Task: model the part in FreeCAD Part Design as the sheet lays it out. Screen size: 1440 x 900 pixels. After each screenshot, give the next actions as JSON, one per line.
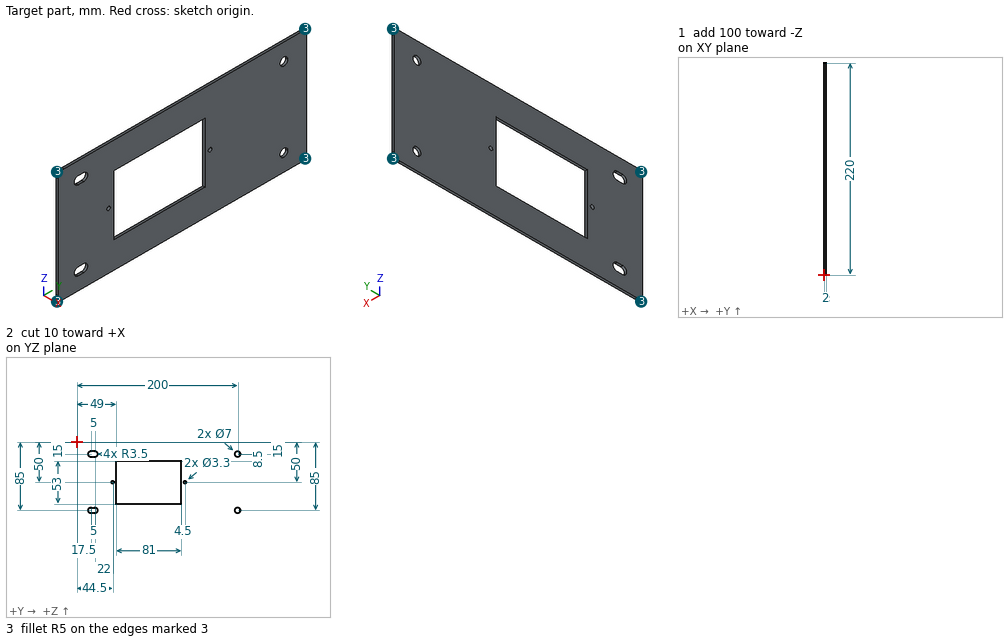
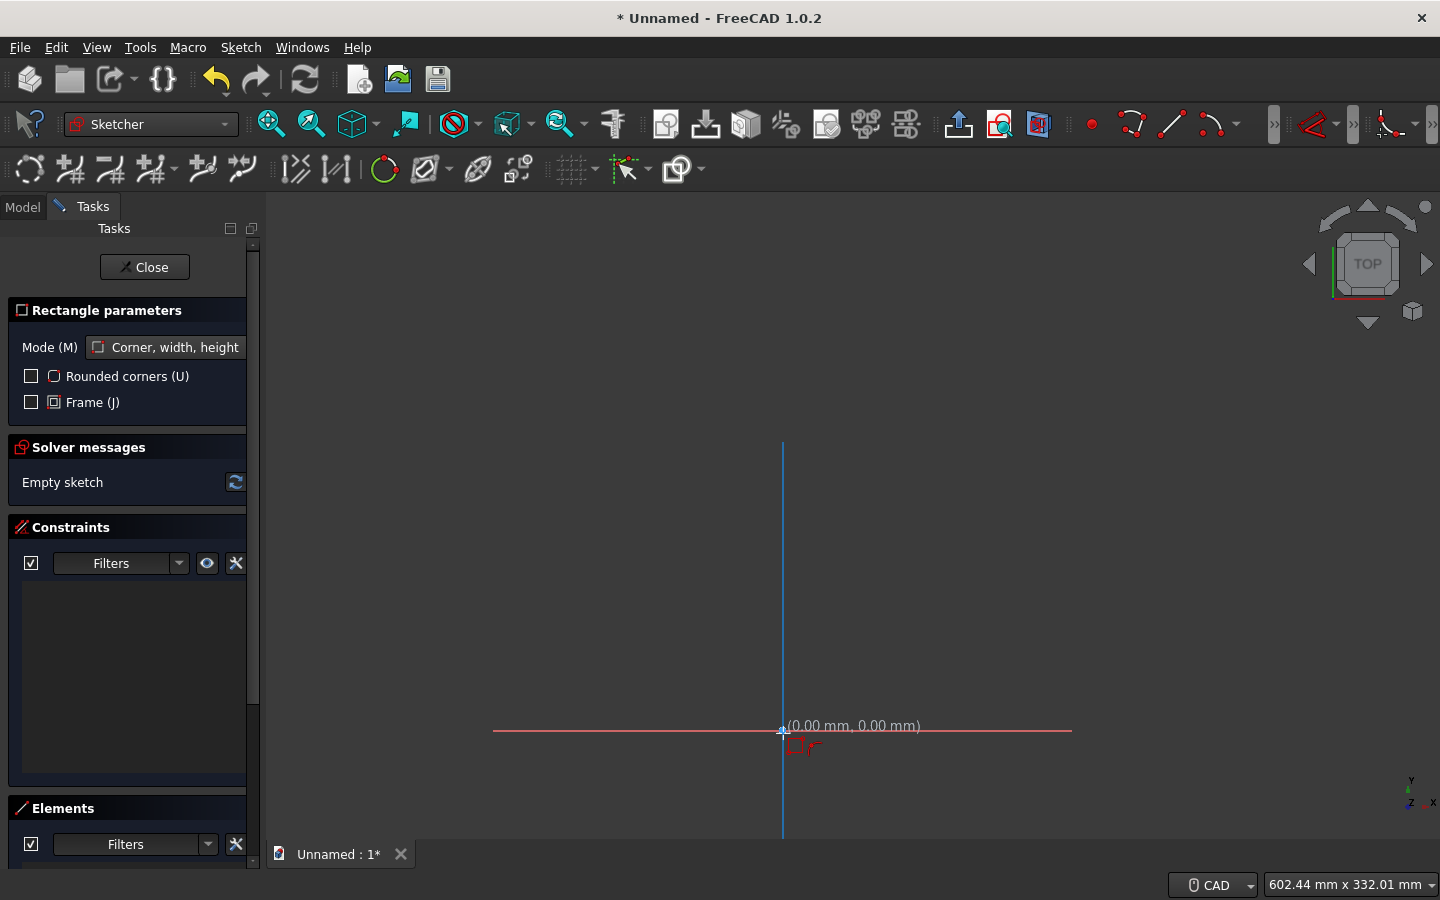
{"action": "left_click", "coordinate": [783, 731]}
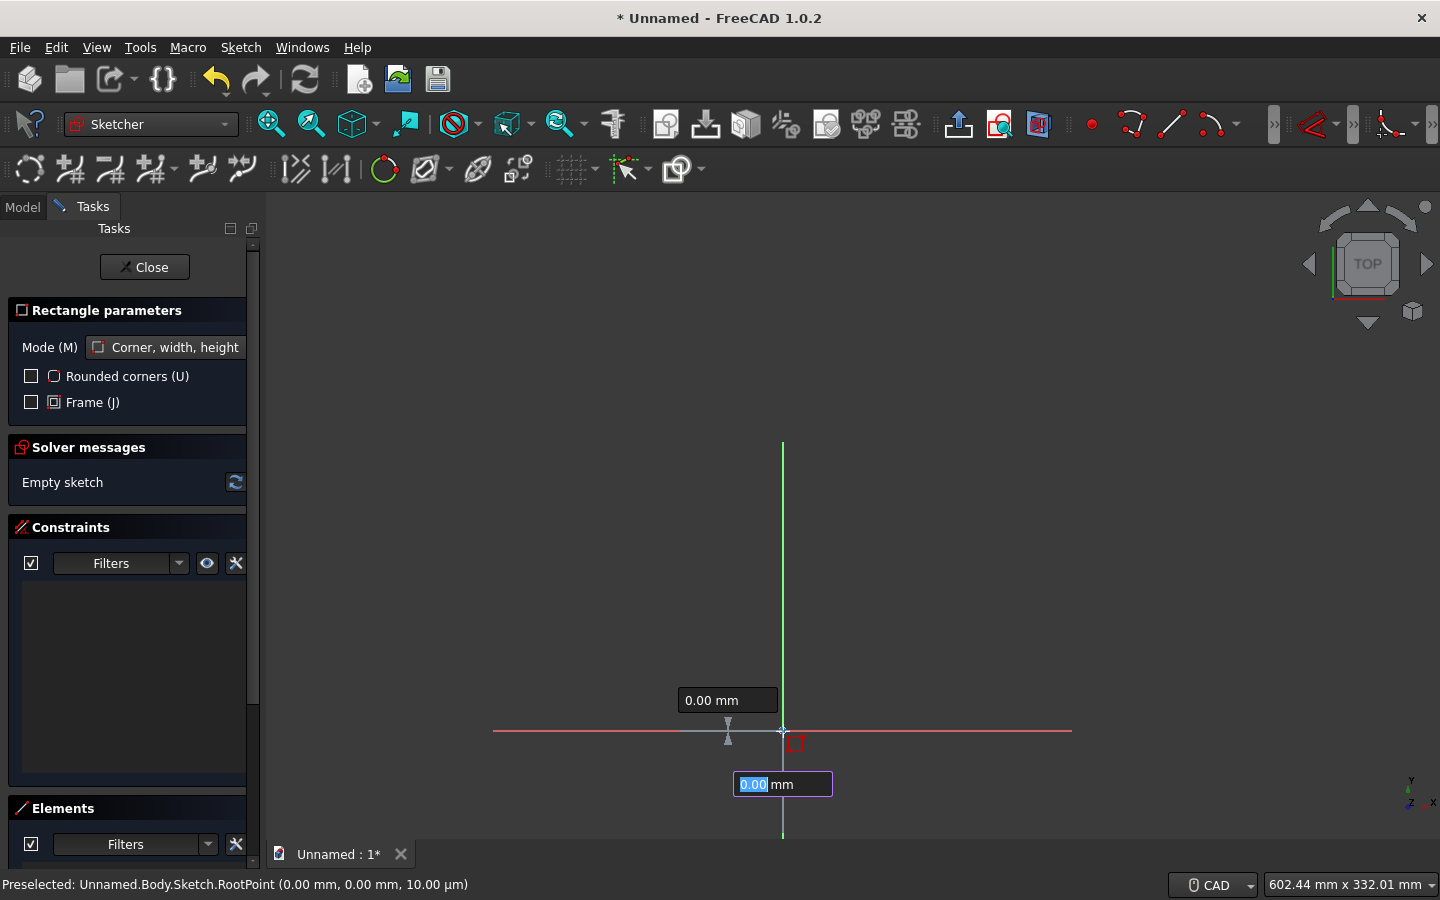
{"action": "scroll", "coordinate": [787, 302], "scroll_direction": "up", "scroll_amount": 8}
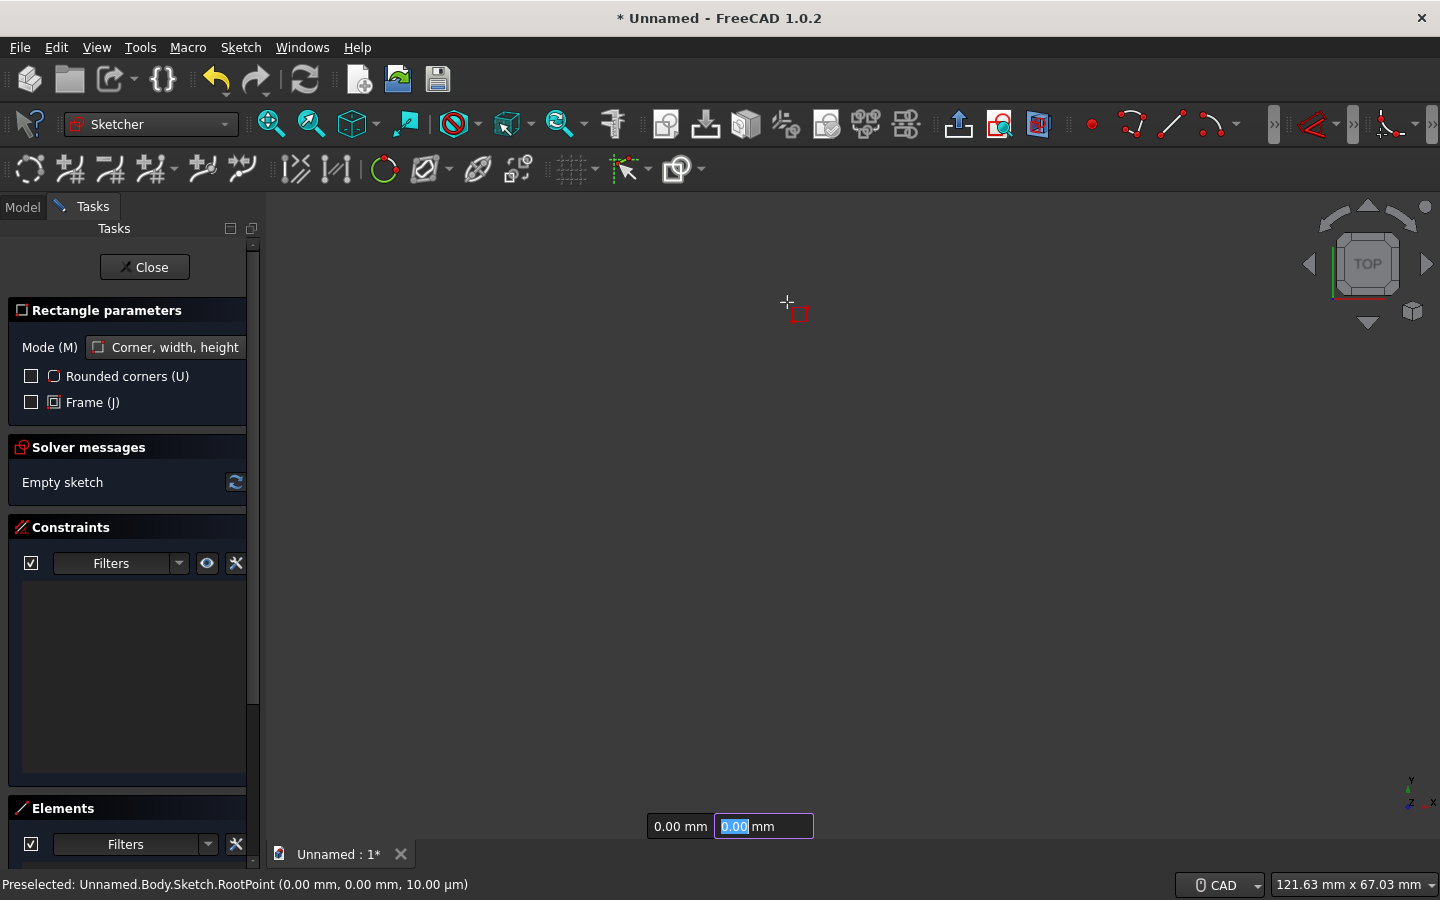
{"action": "left_click", "coordinate": [783, 301]}
{"action": "key", "text": "Escape"}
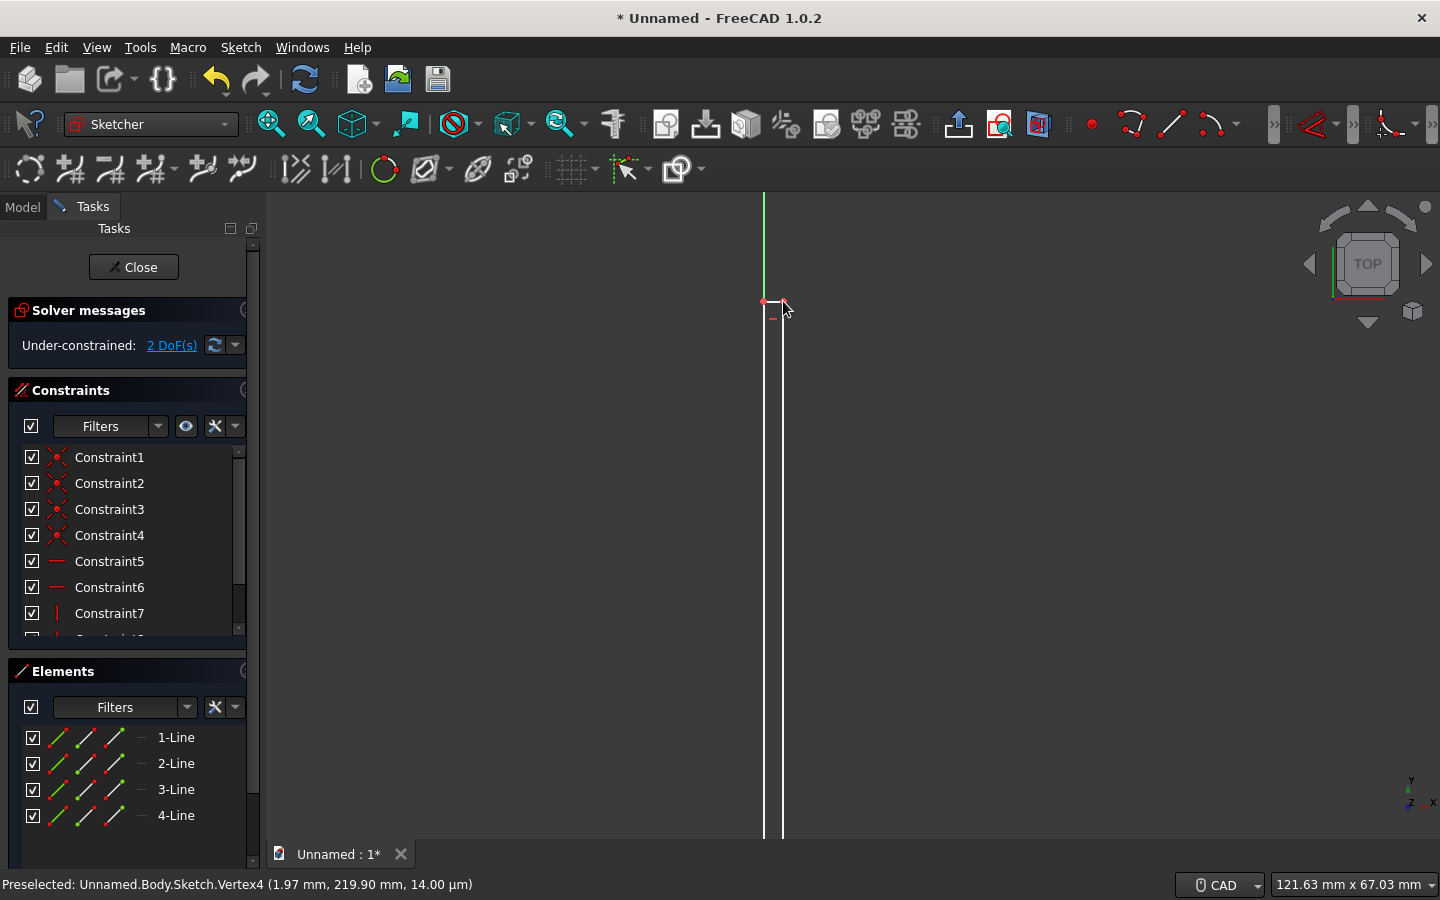
{"action": "scroll", "coordinate": [787, 301], "scroll_direction": "down", "scroll_amount": 8}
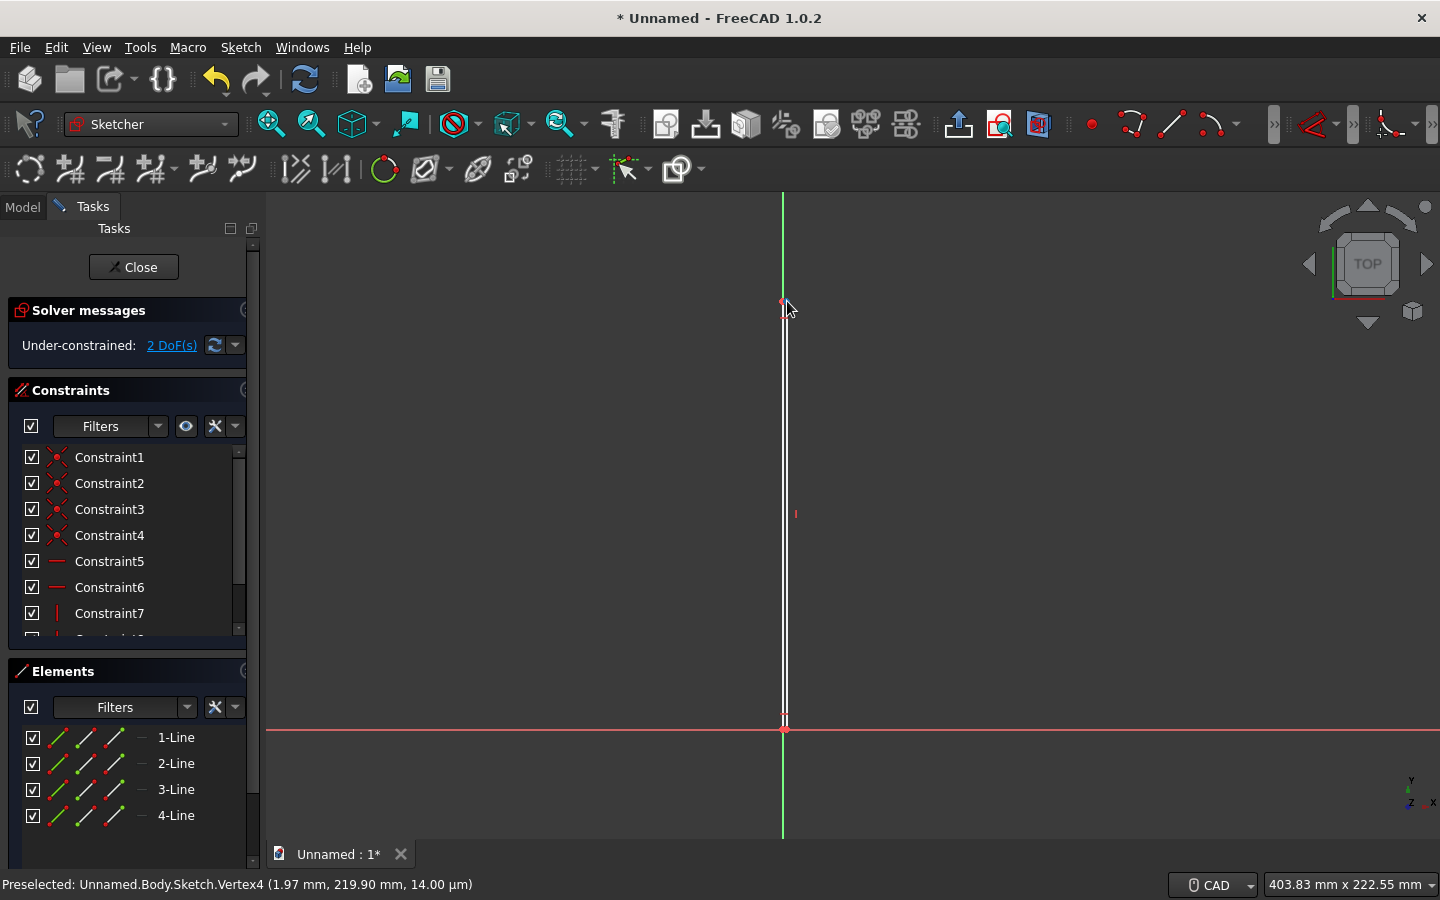
{"action": "scroll", "coordinate": [785, 730], "scroll_direction": "up", "scroll_amount": 12}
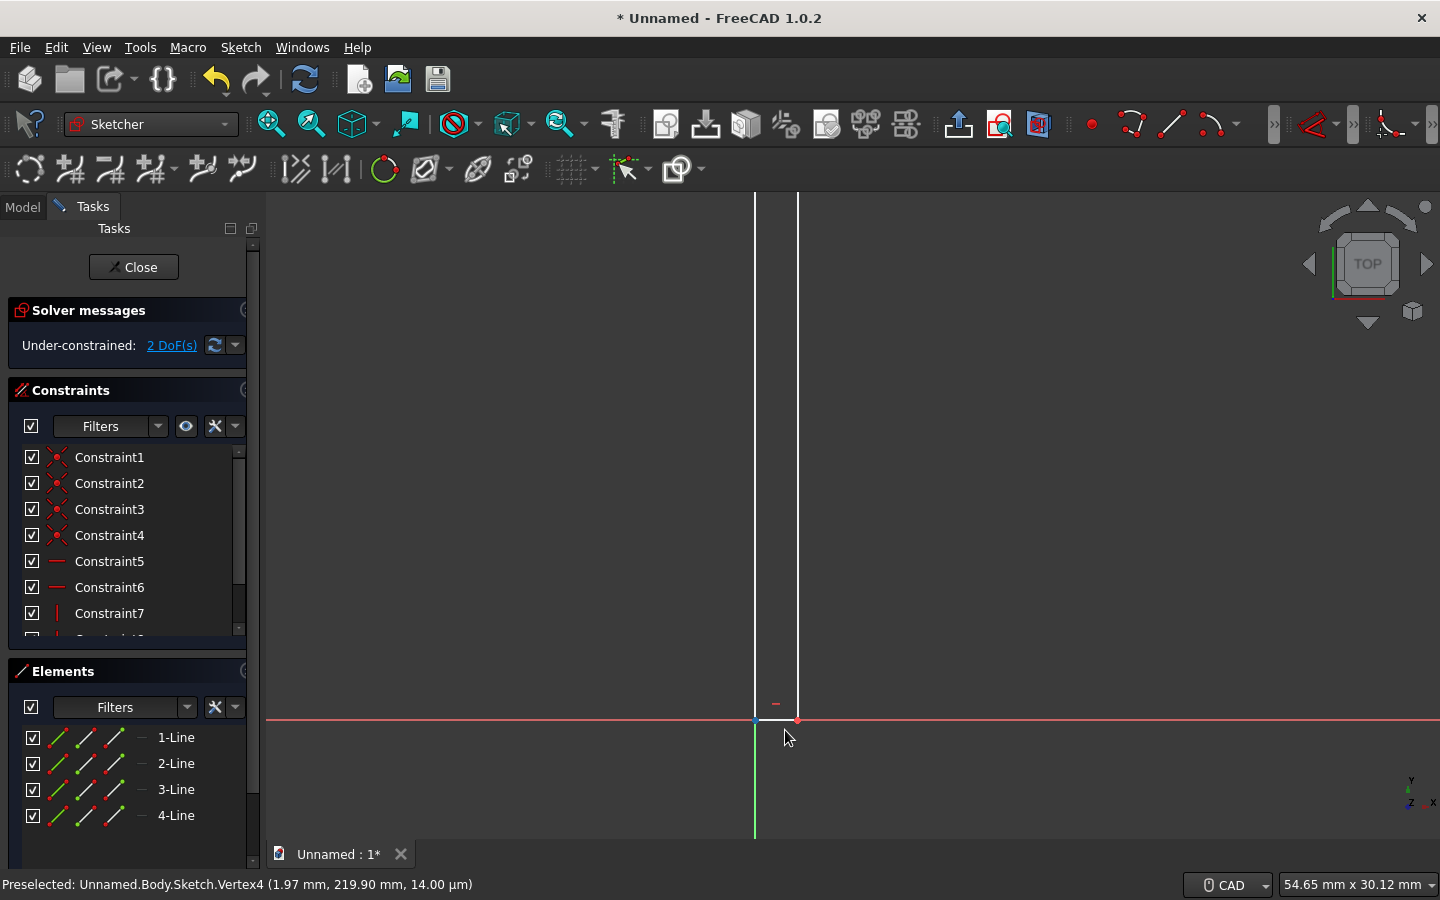
{"action": "left_click", "coordinate": [776, 720]}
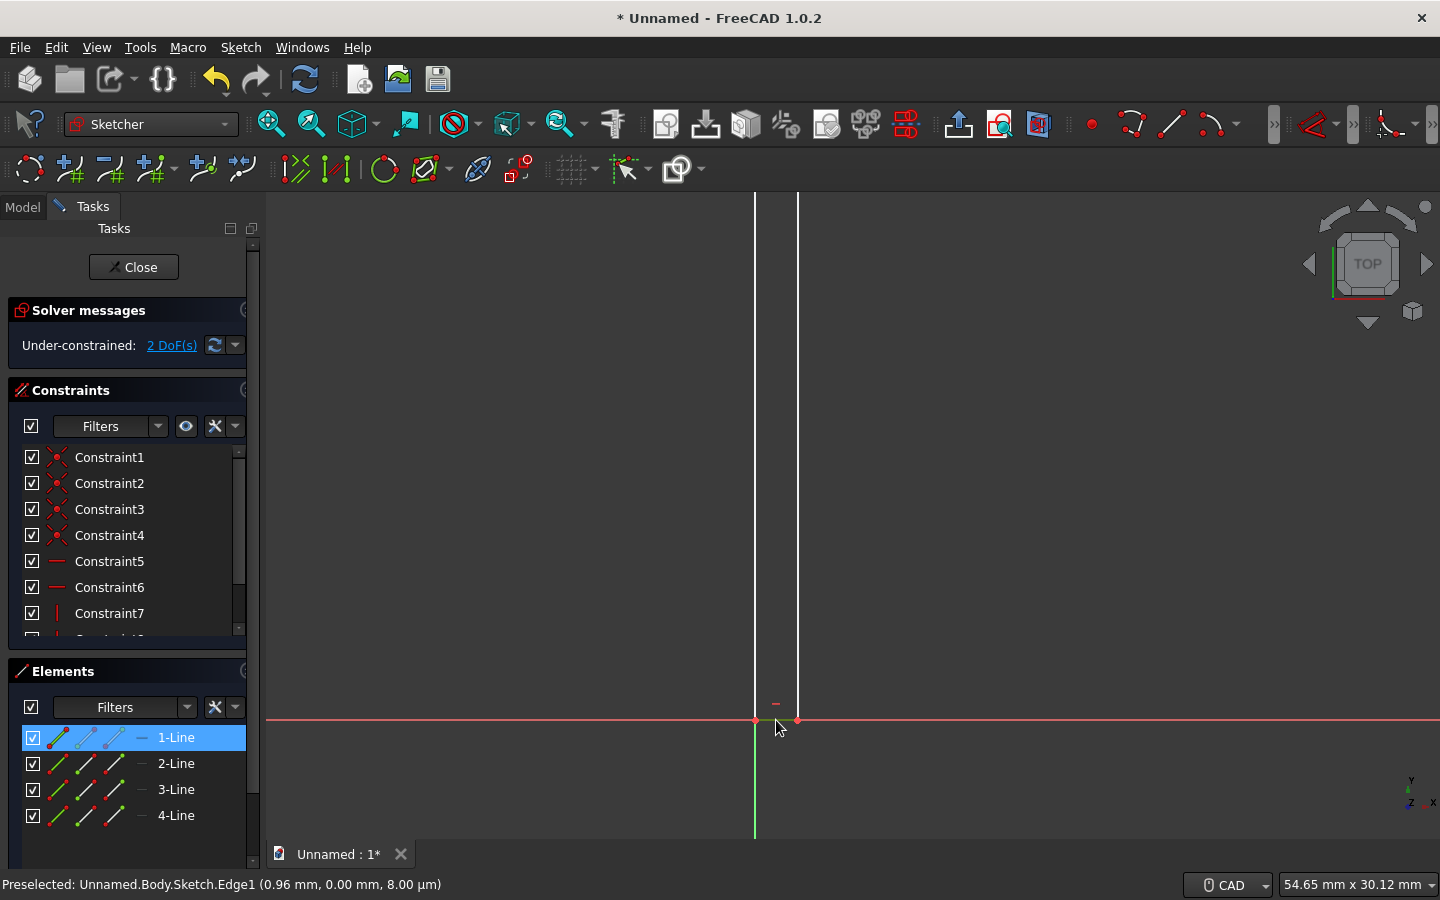
{"action": "left_click", "coordinate": [1338, 124]}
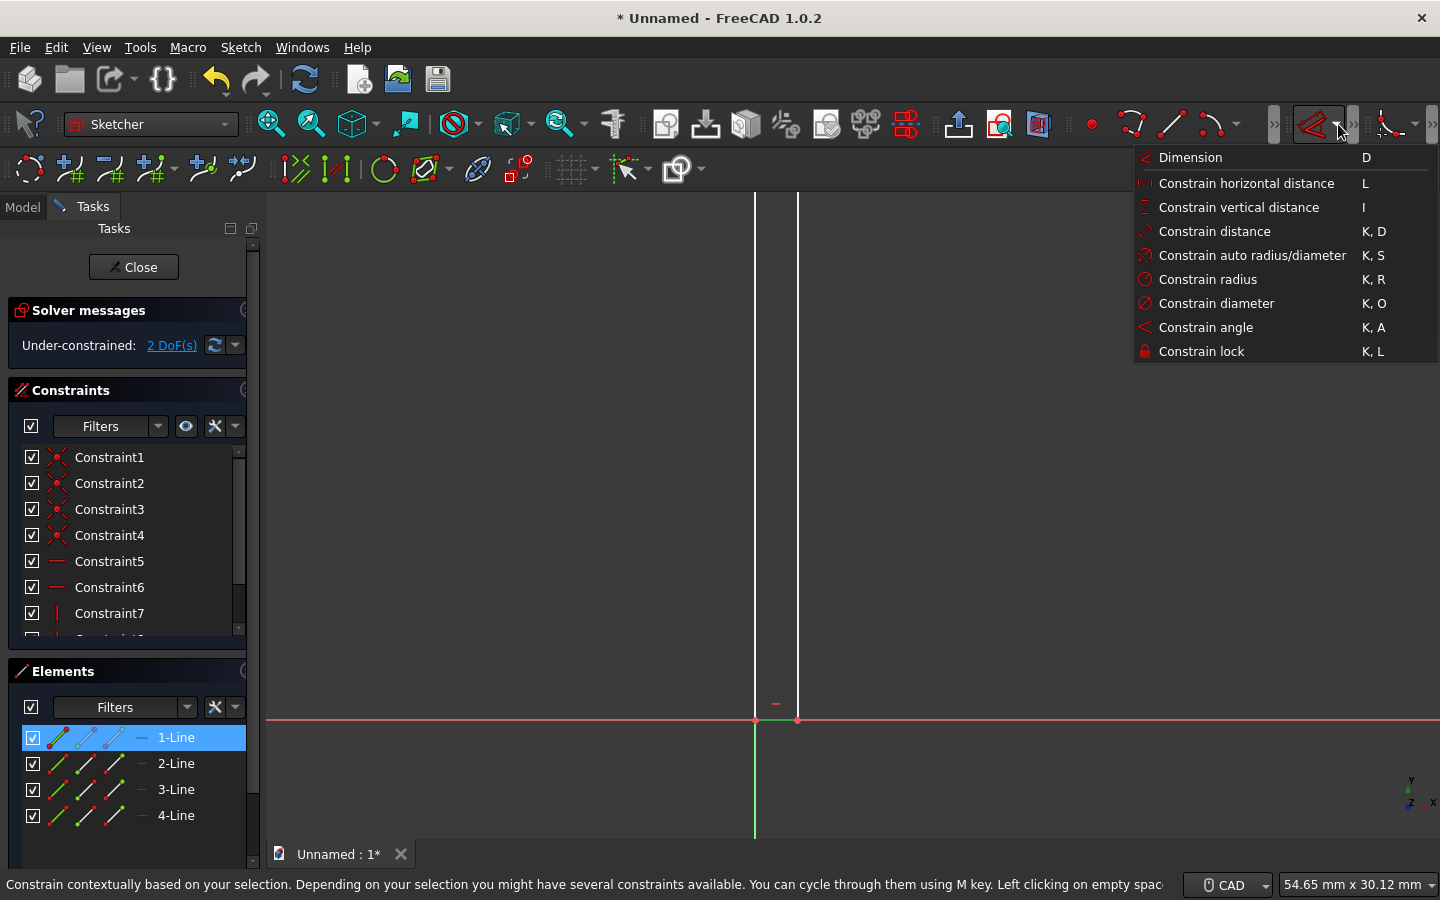
{"action": "left_click", "coordinate": [1286, 183]}